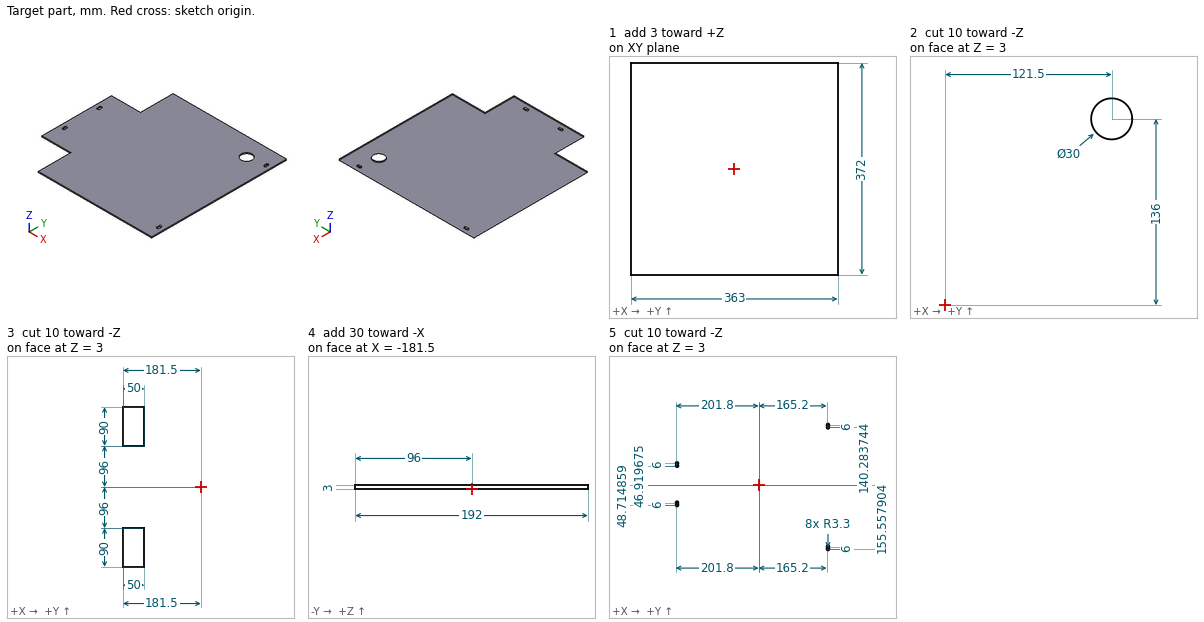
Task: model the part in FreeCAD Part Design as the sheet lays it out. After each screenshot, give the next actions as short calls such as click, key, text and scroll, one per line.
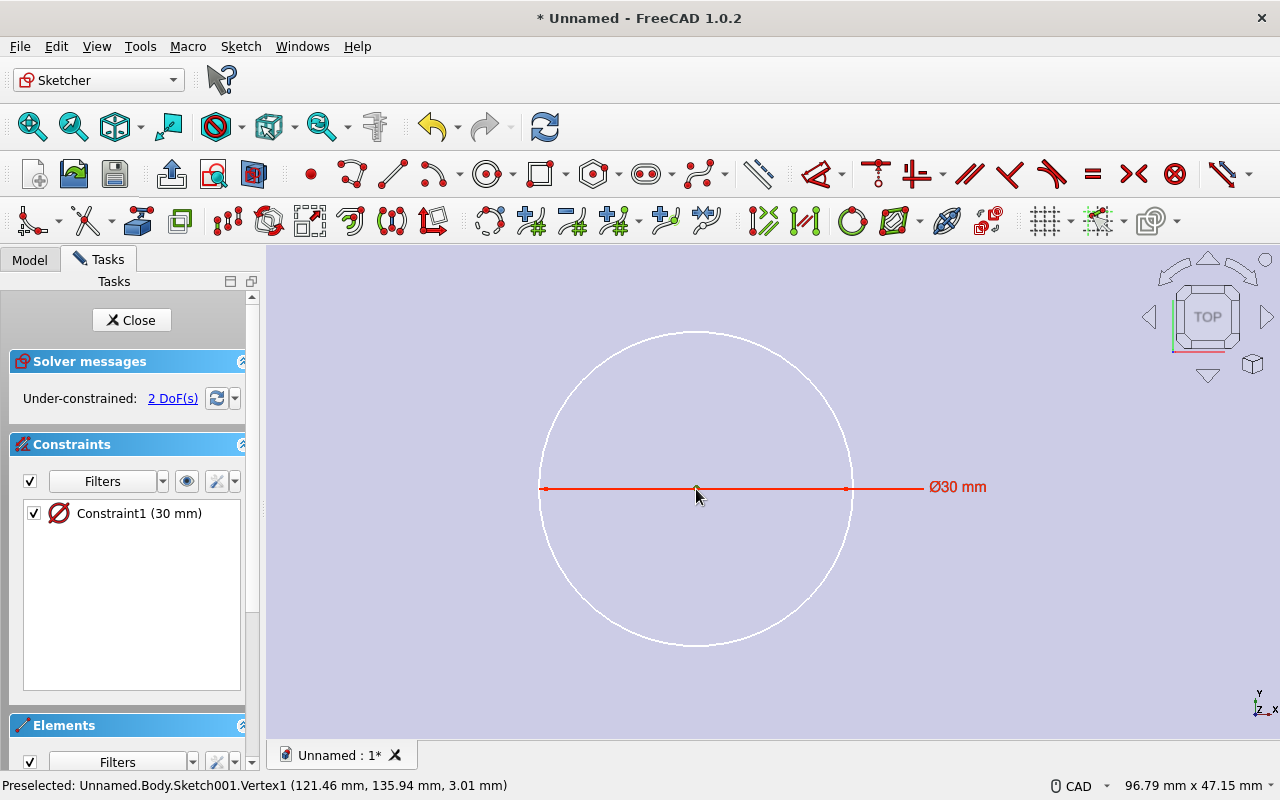
click(842, 174)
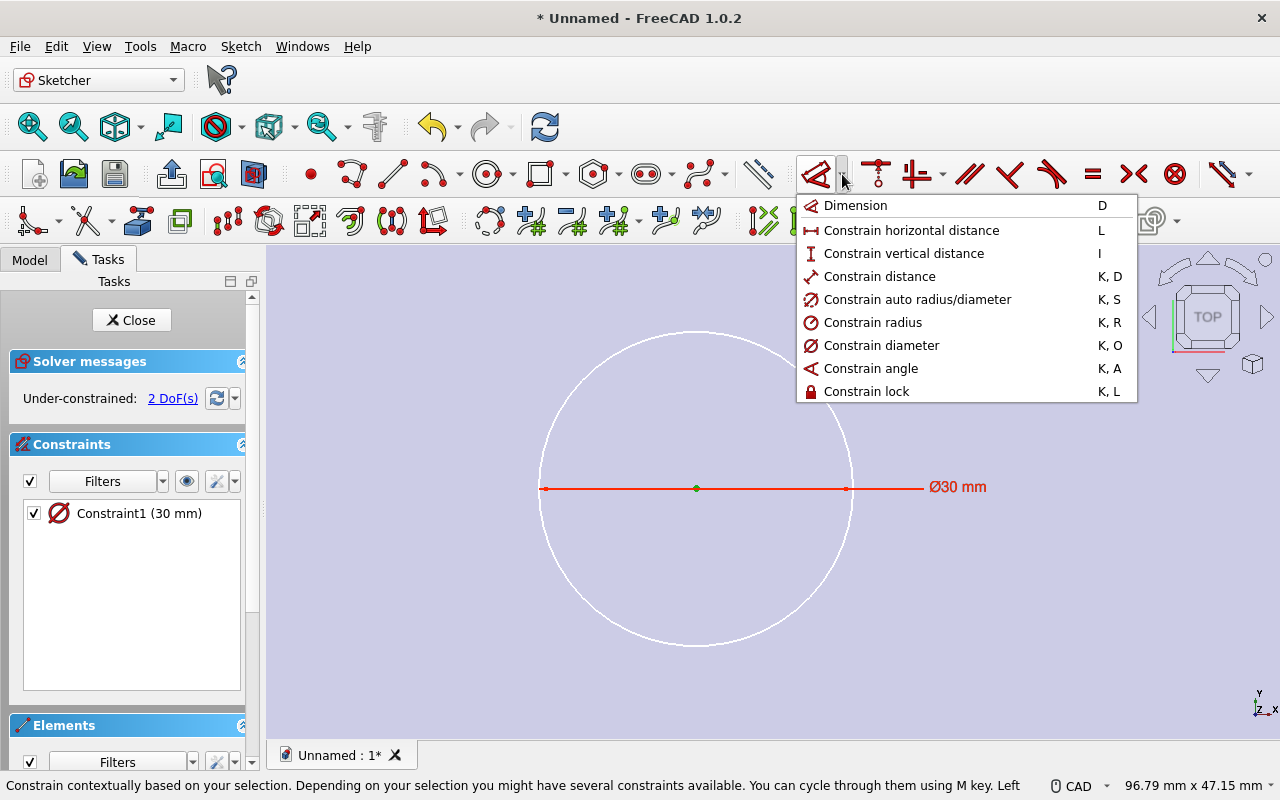
click(967, 254)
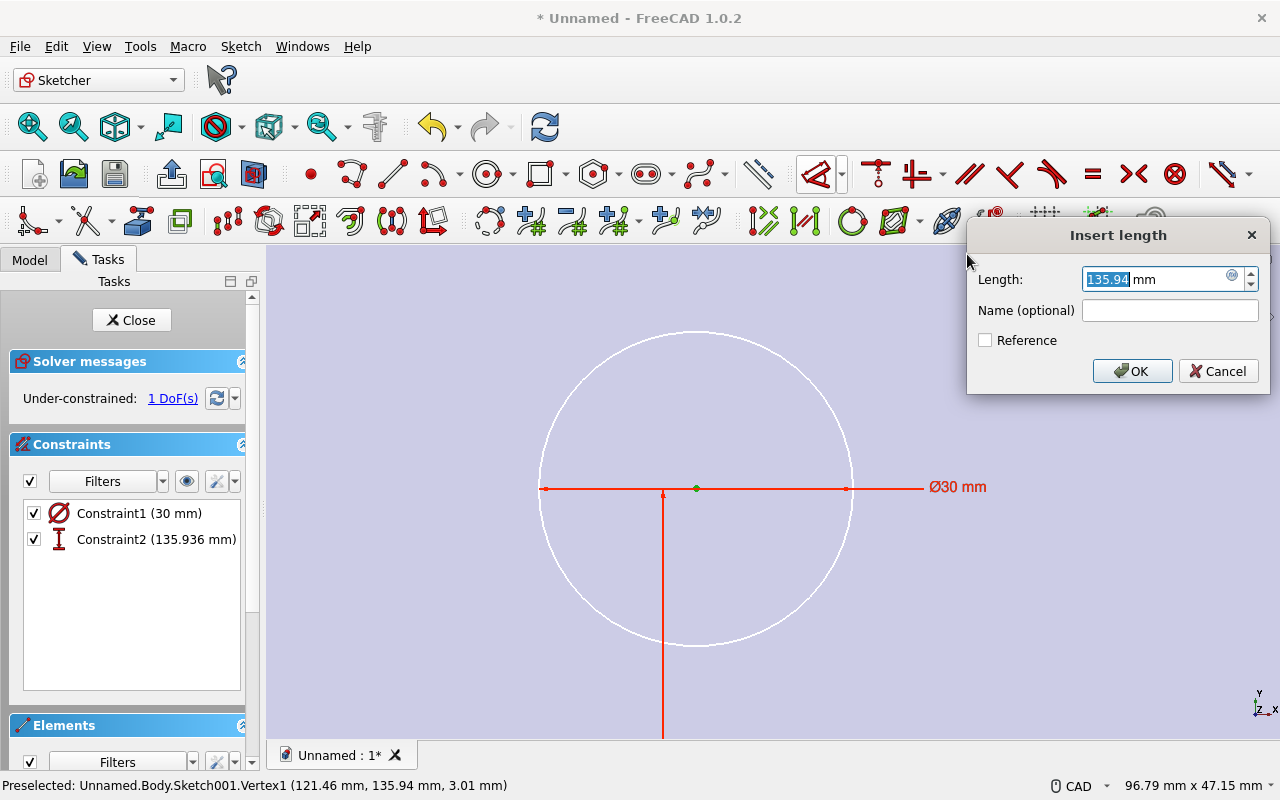
text(136)
key(Return)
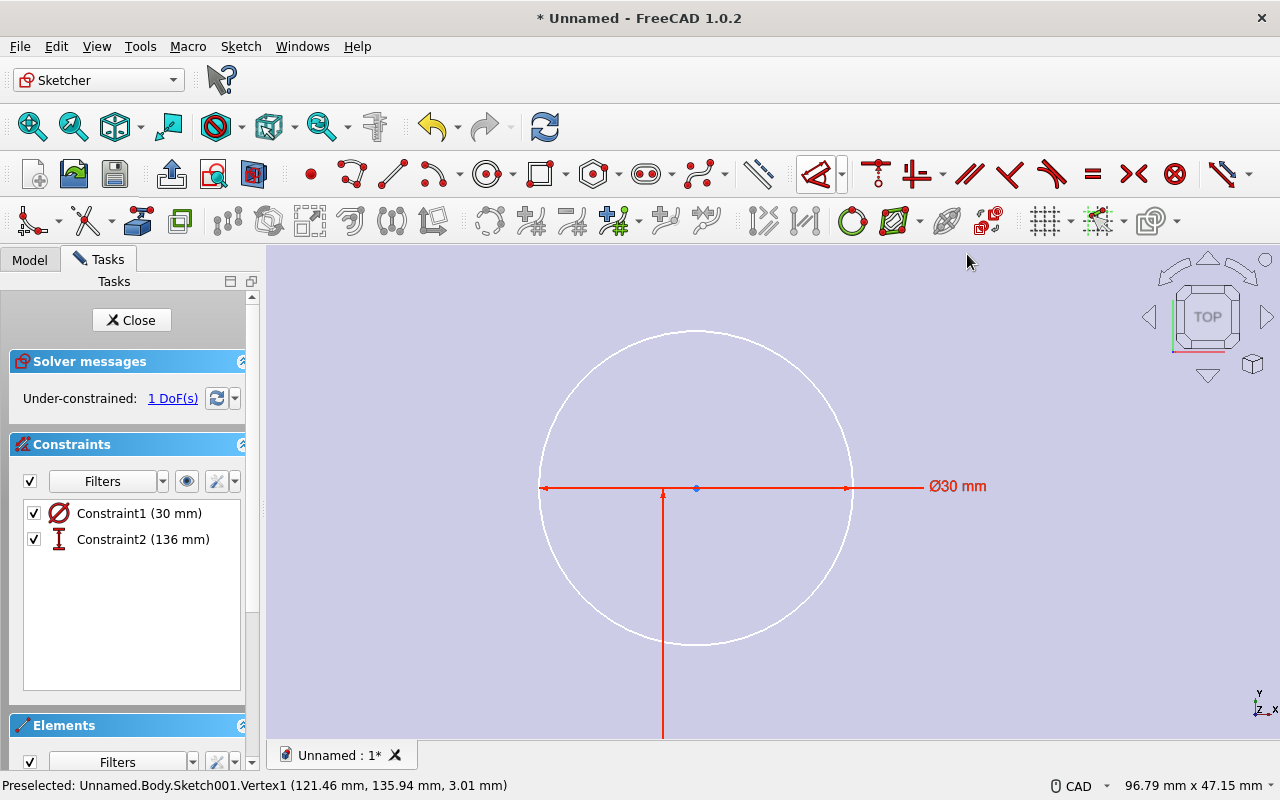
click(696, 488)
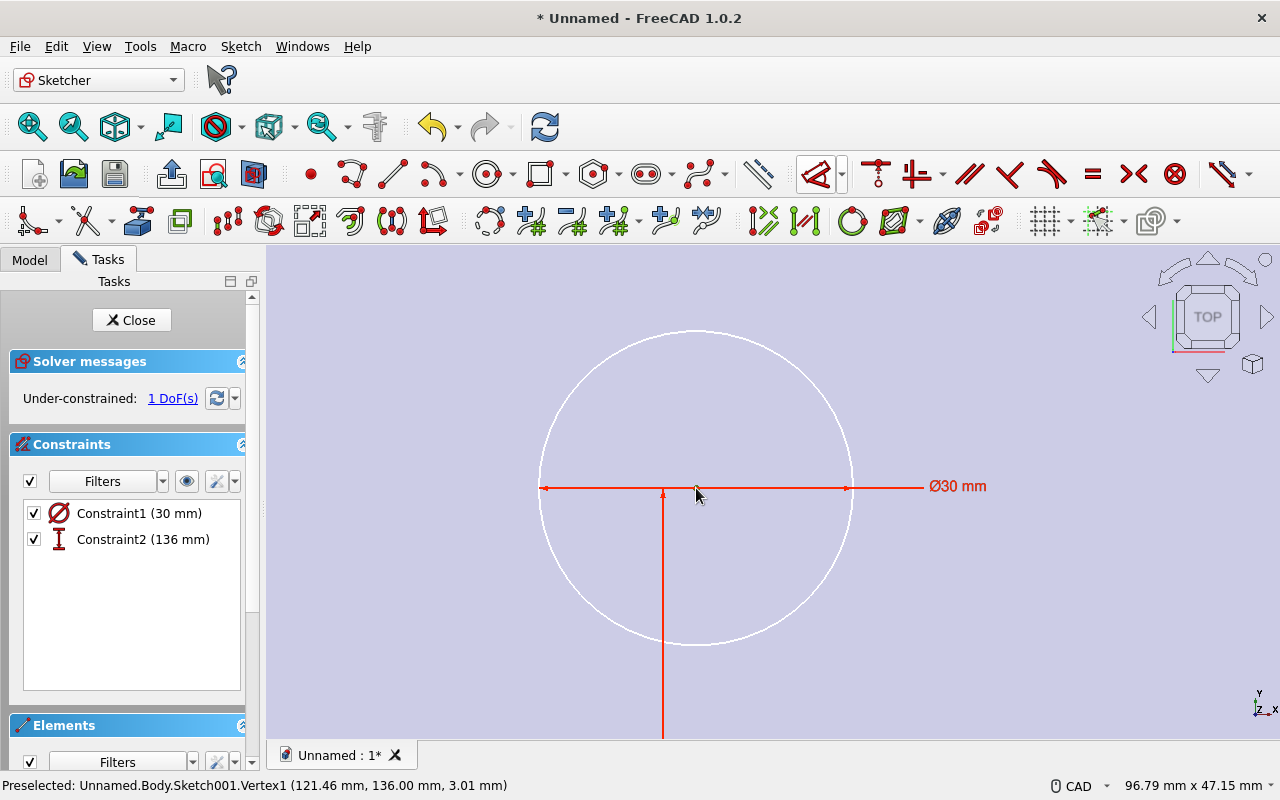
click(842, 174)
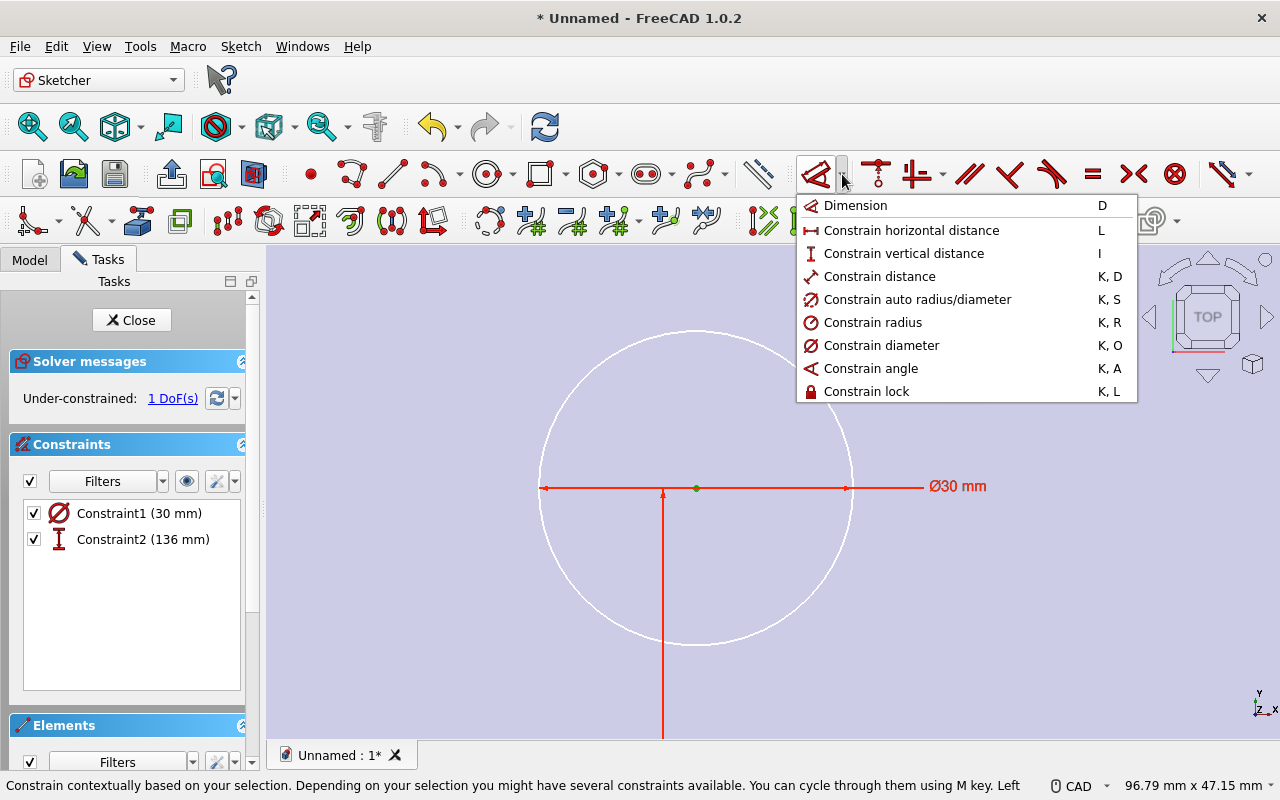
click(967, 230)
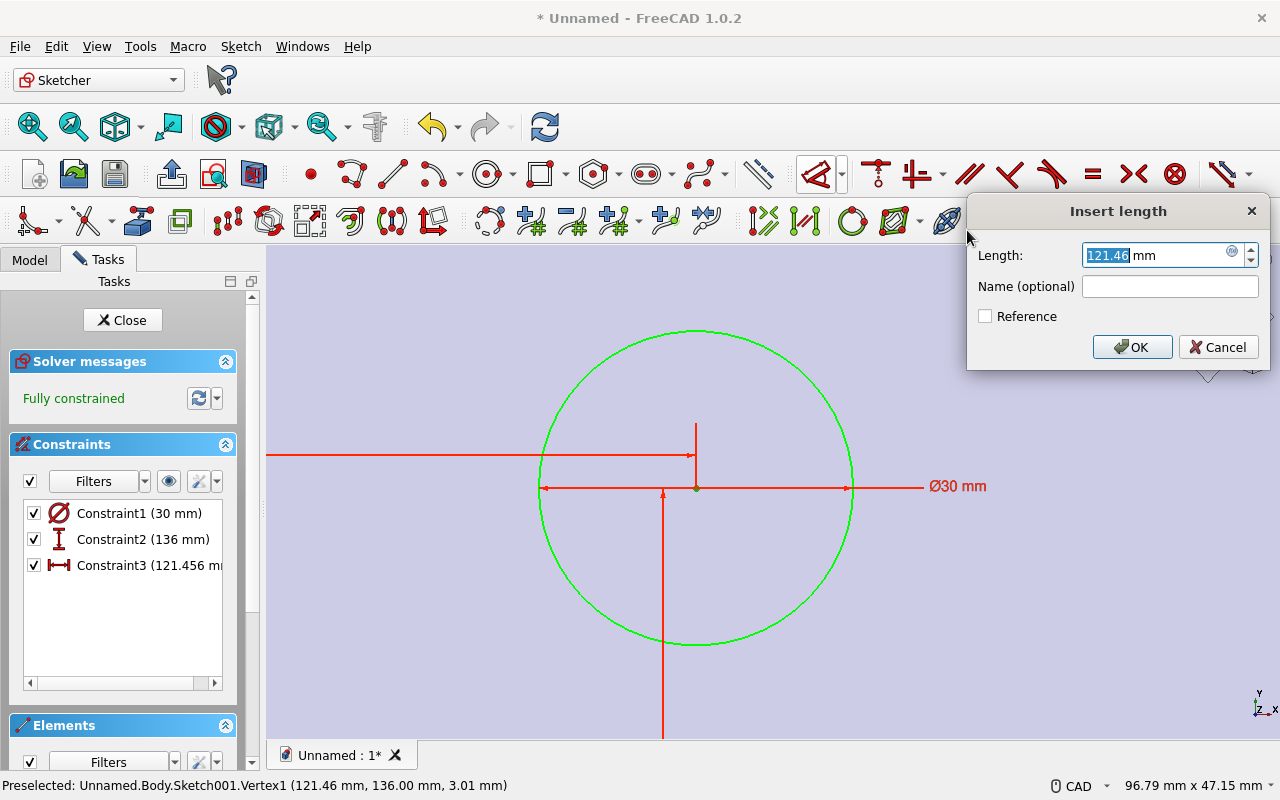
text(121.5)
key(Return)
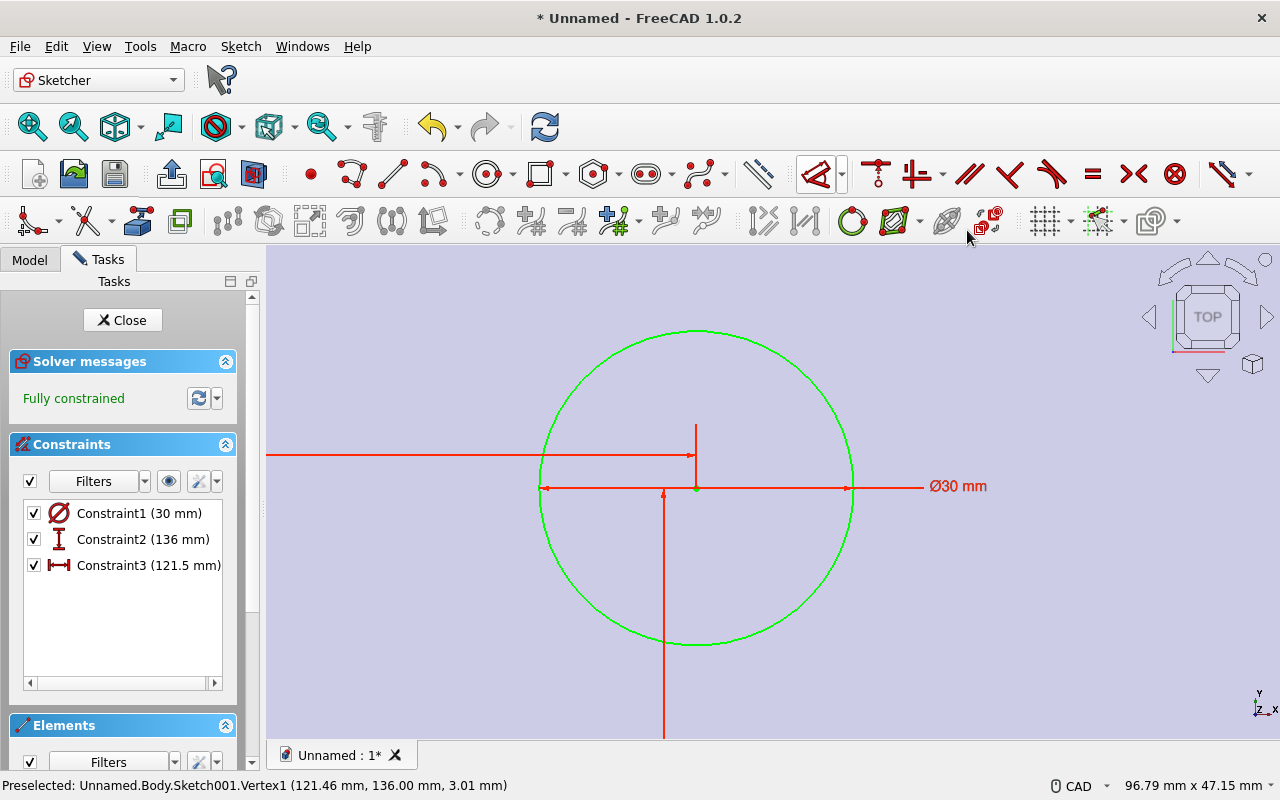
click(123, 320)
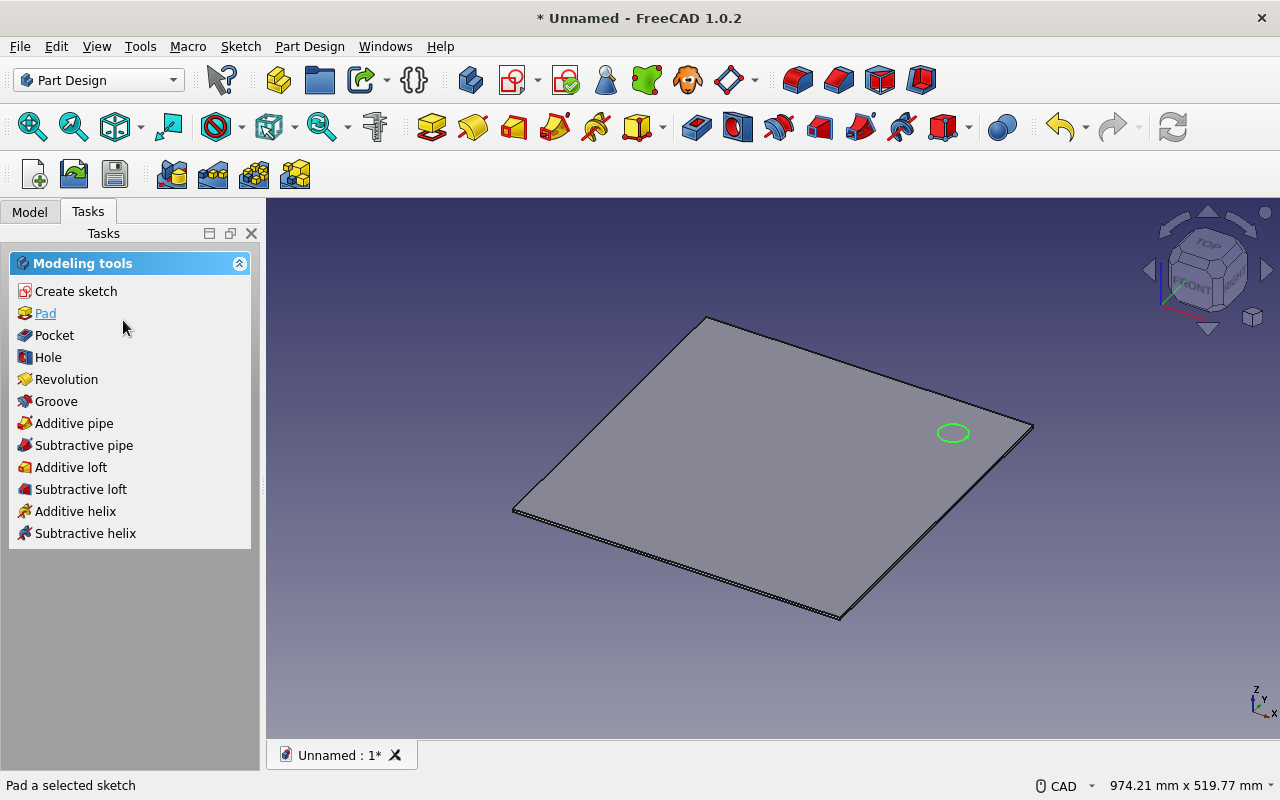
click(697, 128)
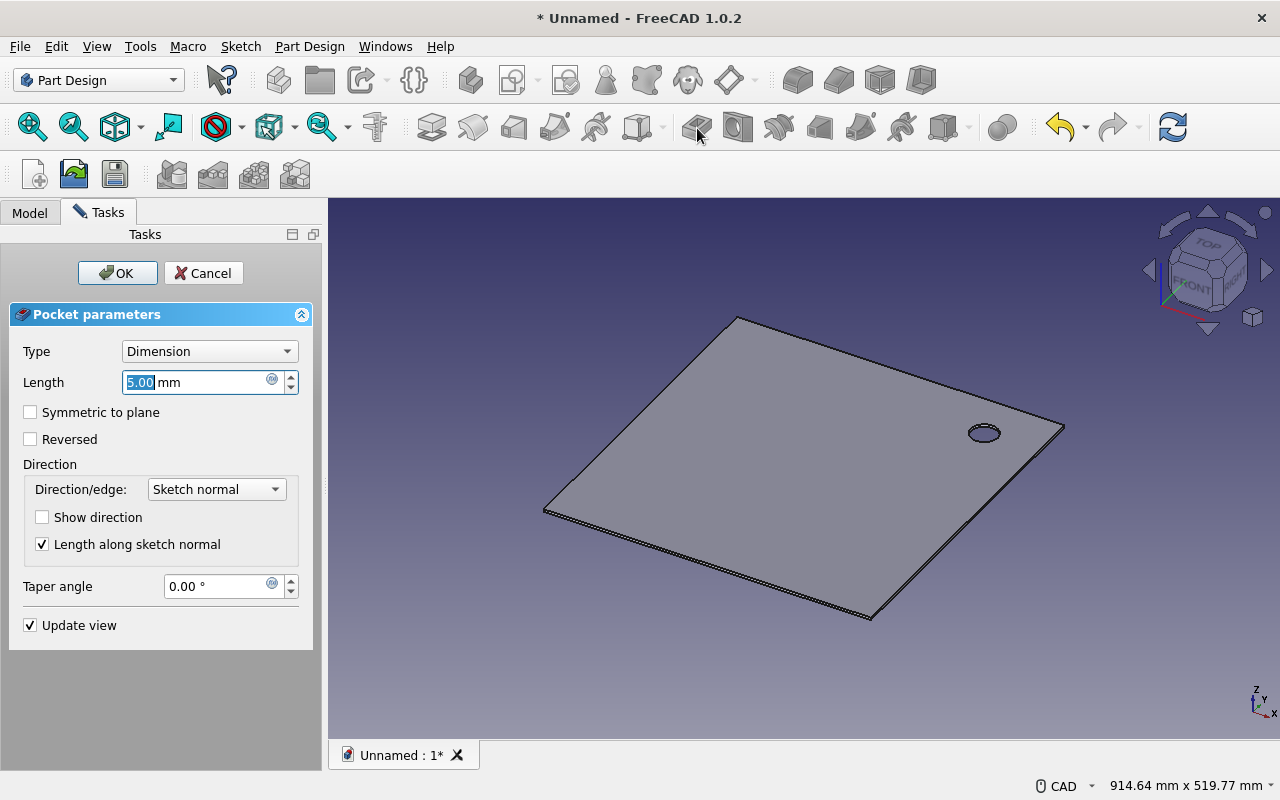
text(10)
key(Tab)